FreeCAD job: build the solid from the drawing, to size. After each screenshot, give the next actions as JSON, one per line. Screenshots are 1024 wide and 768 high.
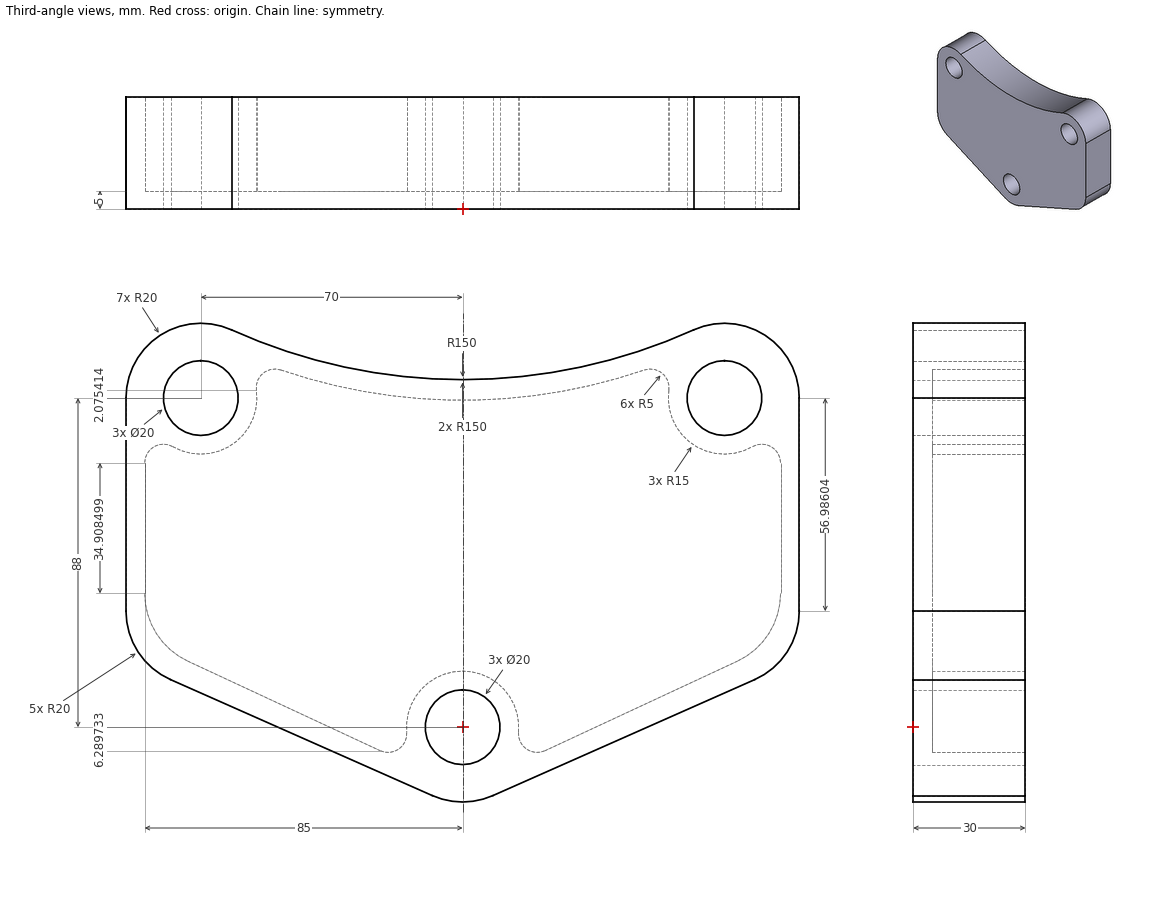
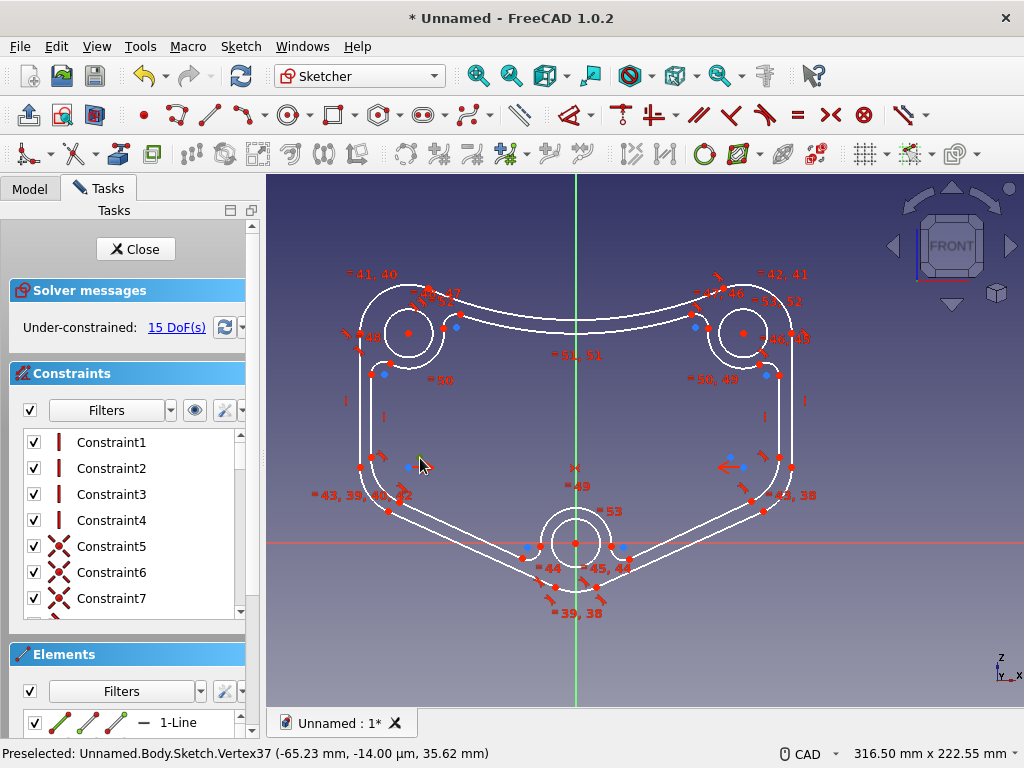
{"action": "left_click", "coordinate": [730, 458]}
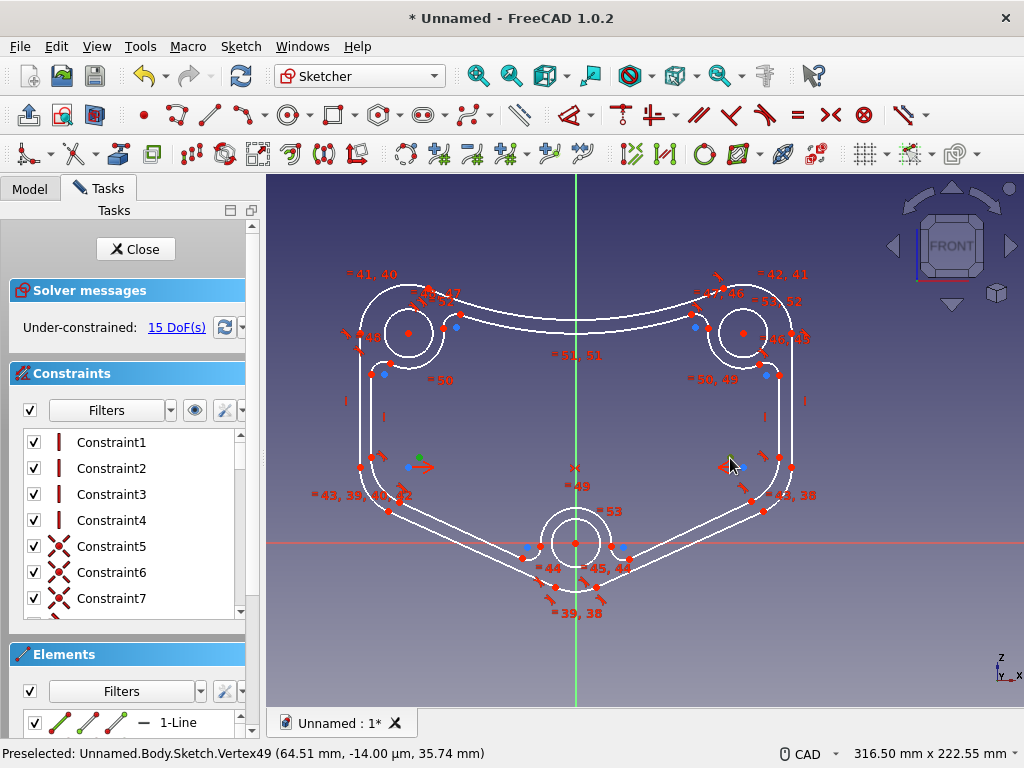
{"action": "left_click", "coordinate": [576, 645]}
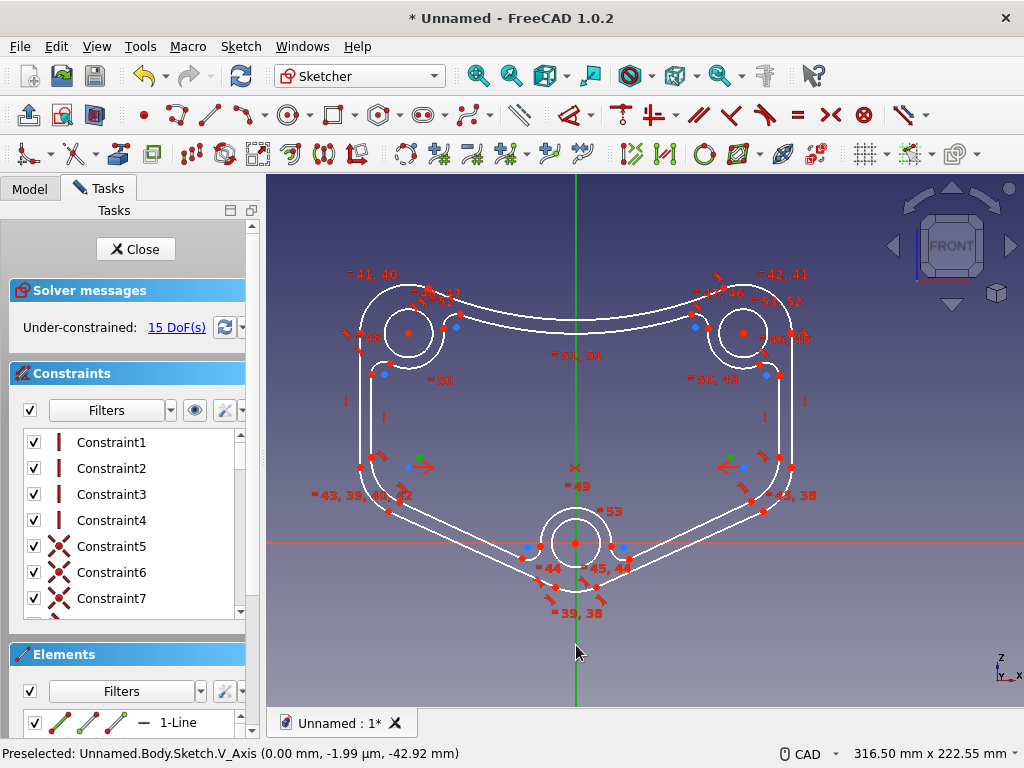
{"action": "left_click", "coordinate": [831, 116]}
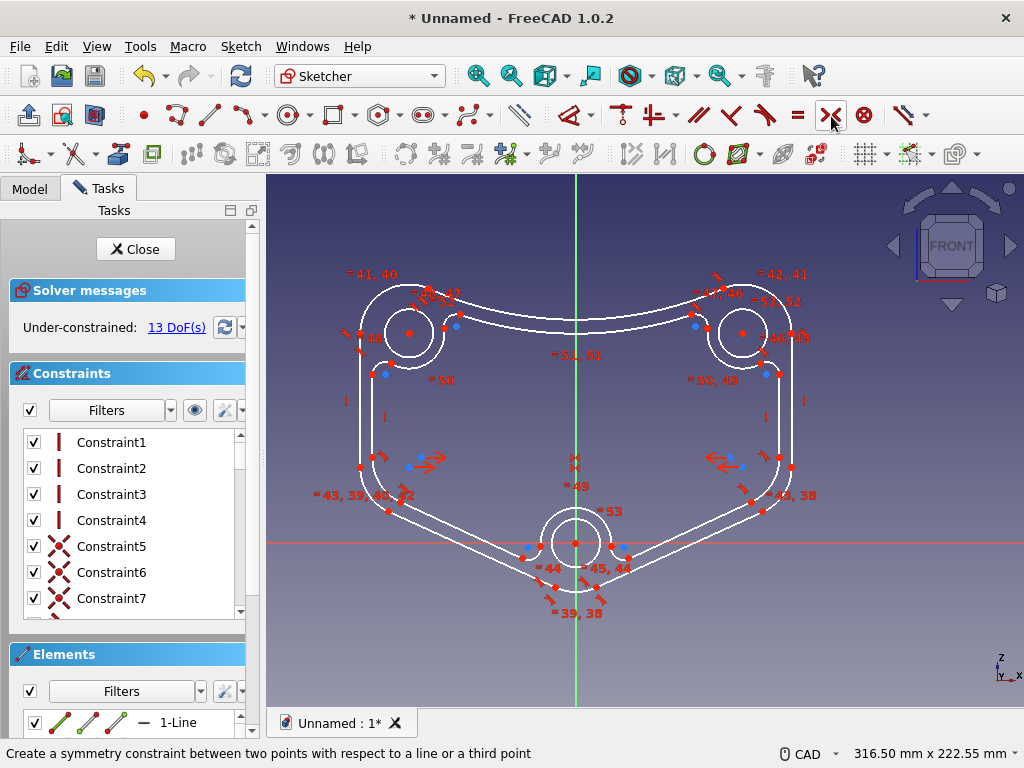
{"action": "left_click", "coordinate": [568, 116]}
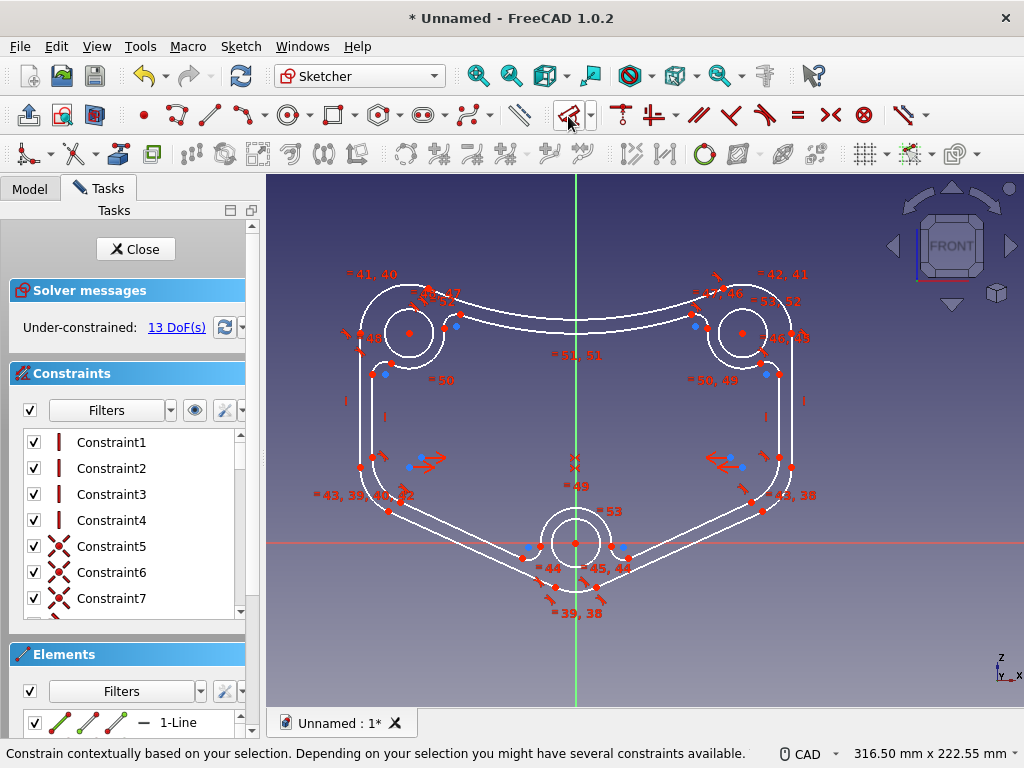
{"action": "left_click", "coordinate": [777, 502]}
{"action": "left_click", "coordinate": [800, 525]}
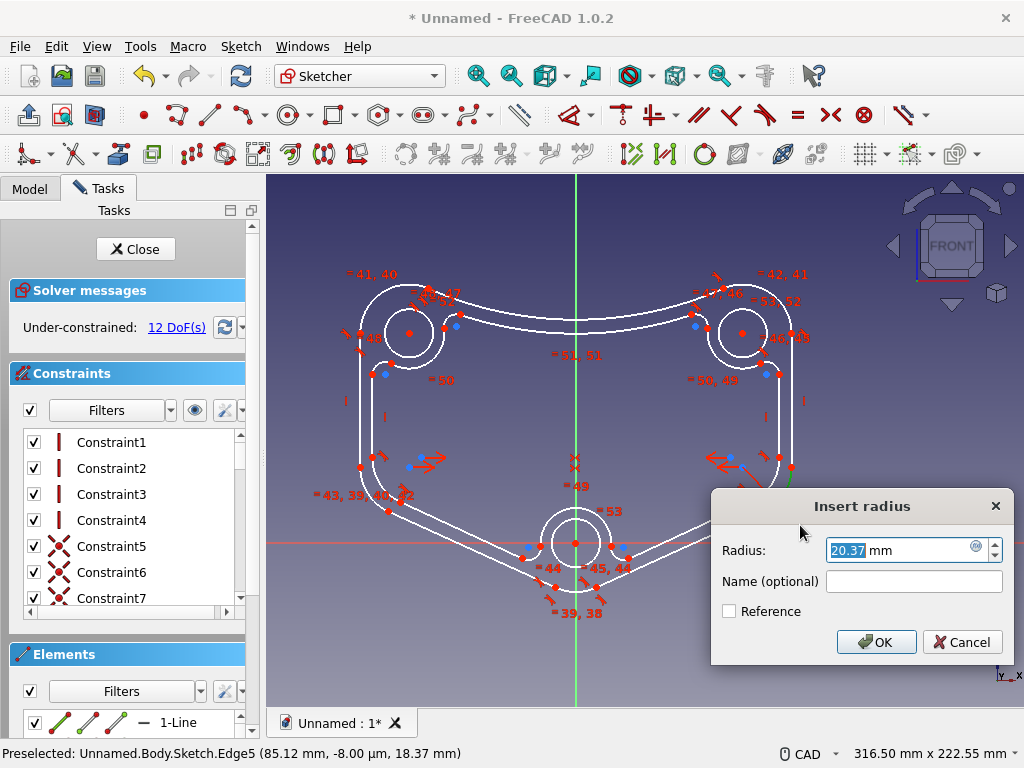
{"action": "type", "text": "20"}
{"action": "key", "text": "Return"}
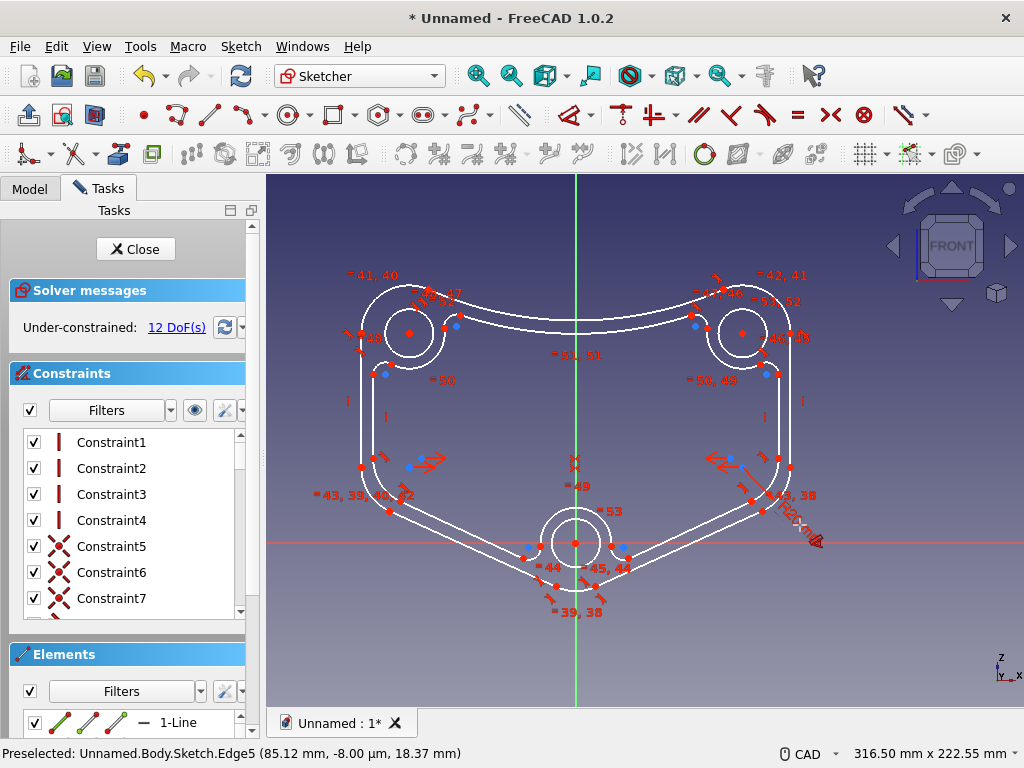
{"action": "left_click", "coordinate": [516, 315]}
{"action": "left_click", "coordinate": [511, 347]}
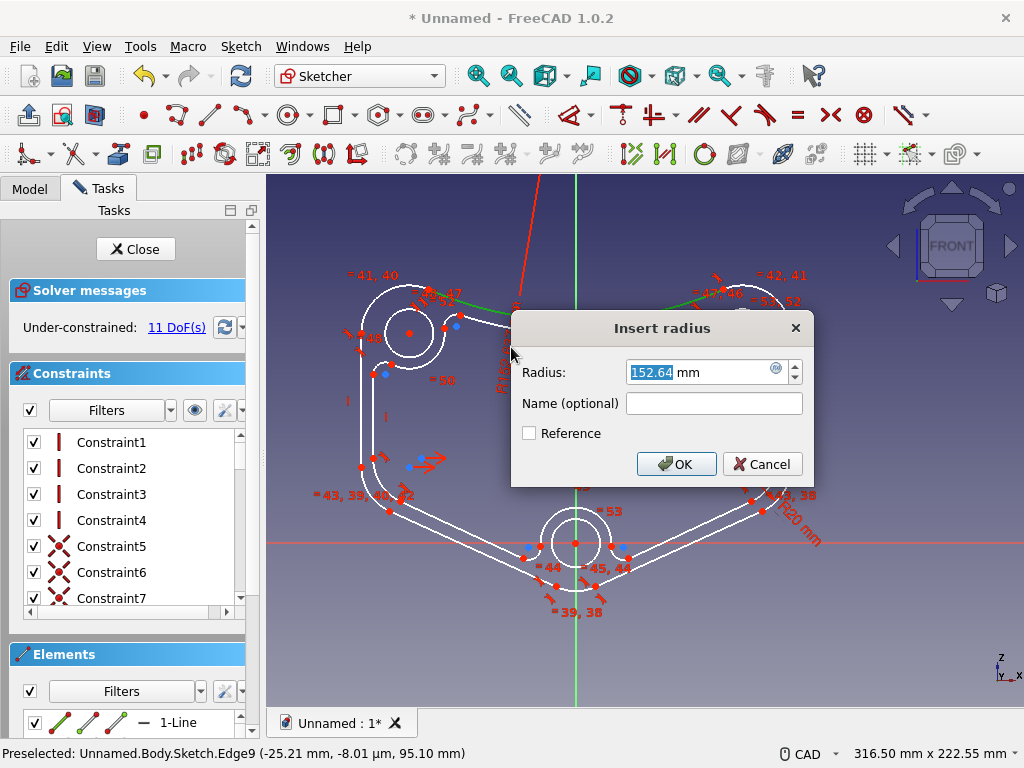
{"action": "type", "text": "150"}
{"action": "key", "text": "Return"}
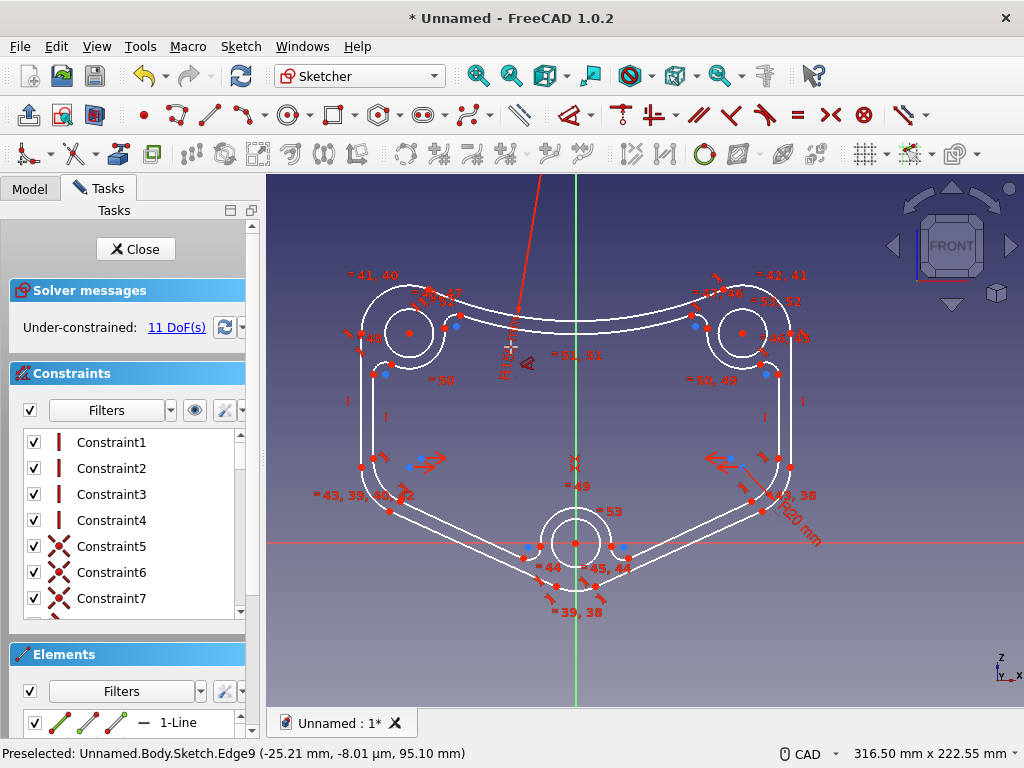
{"action": "scroll", "coordinate": [535, 558], "scroll_direction": "up", "scroll_amount": 6}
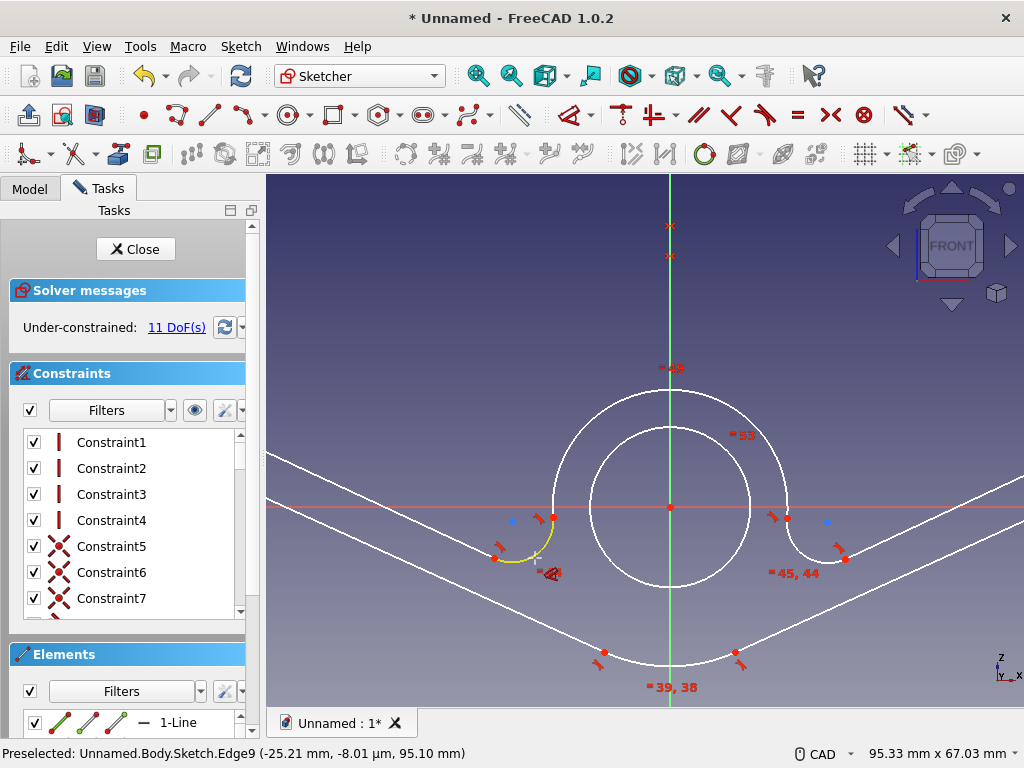
{"action": "left_click", "coordinate": [536, 555]}
{"action": "left_click", "coordinate": [554, 581]}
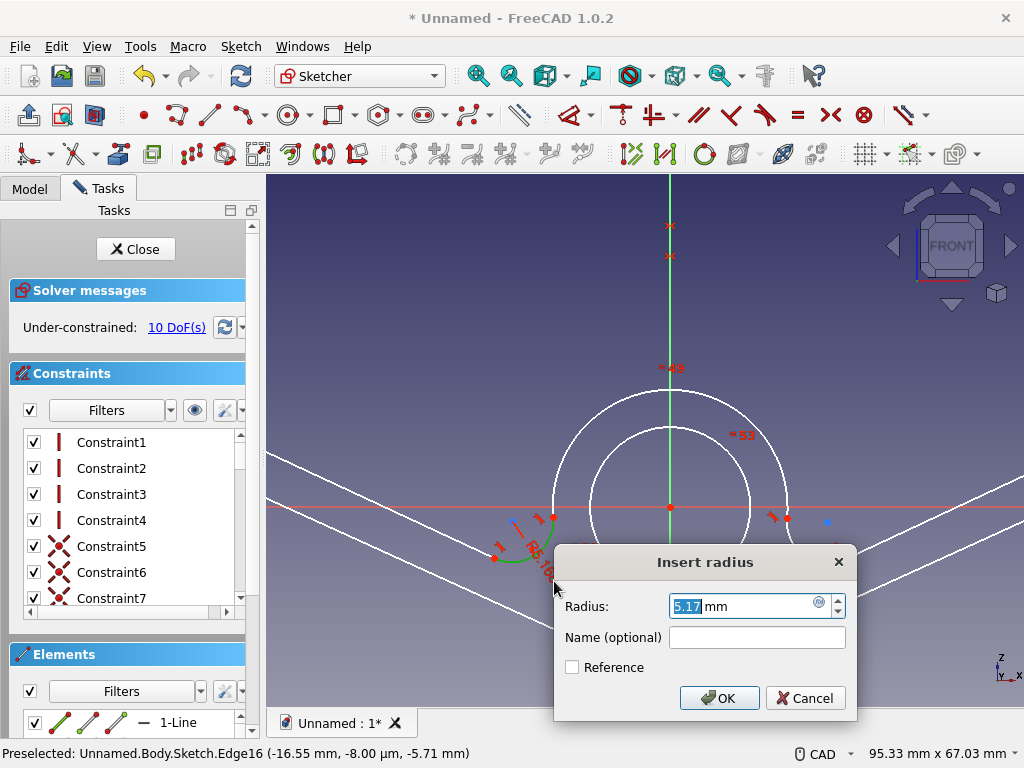
{"action": "type", "text": "5"}
{"action": "key", "text": "Return"}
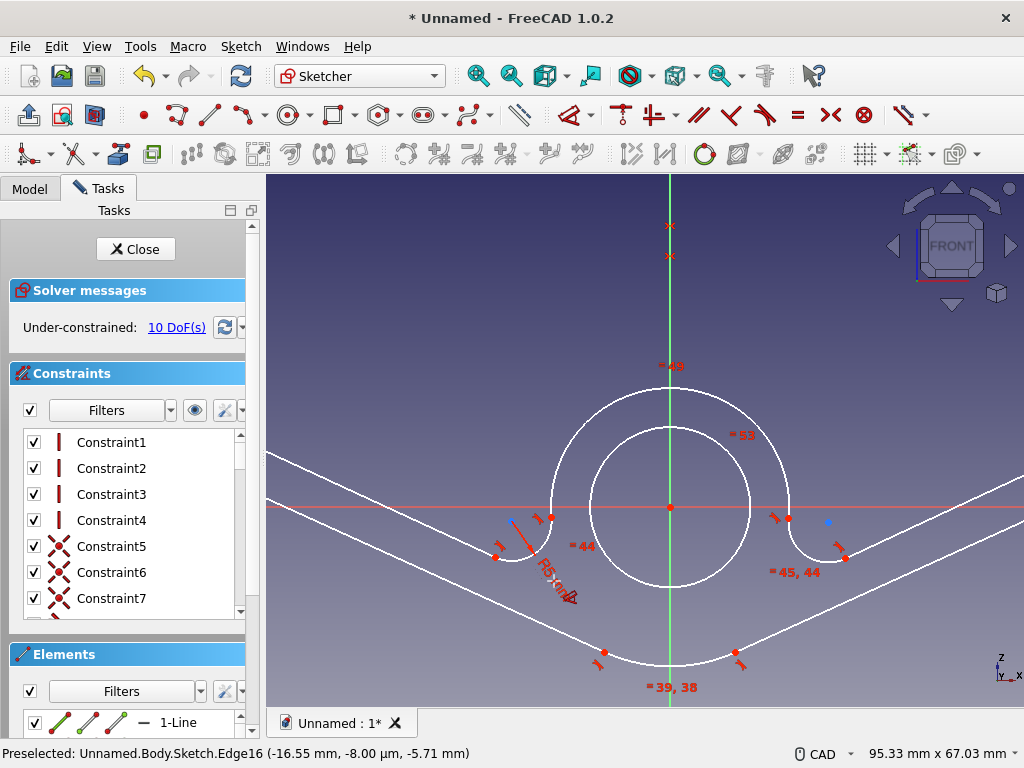
{"action": "left_click", "coordinate": [744, 414]}
{"action": "left_click", "coordinate": [764, 389]}